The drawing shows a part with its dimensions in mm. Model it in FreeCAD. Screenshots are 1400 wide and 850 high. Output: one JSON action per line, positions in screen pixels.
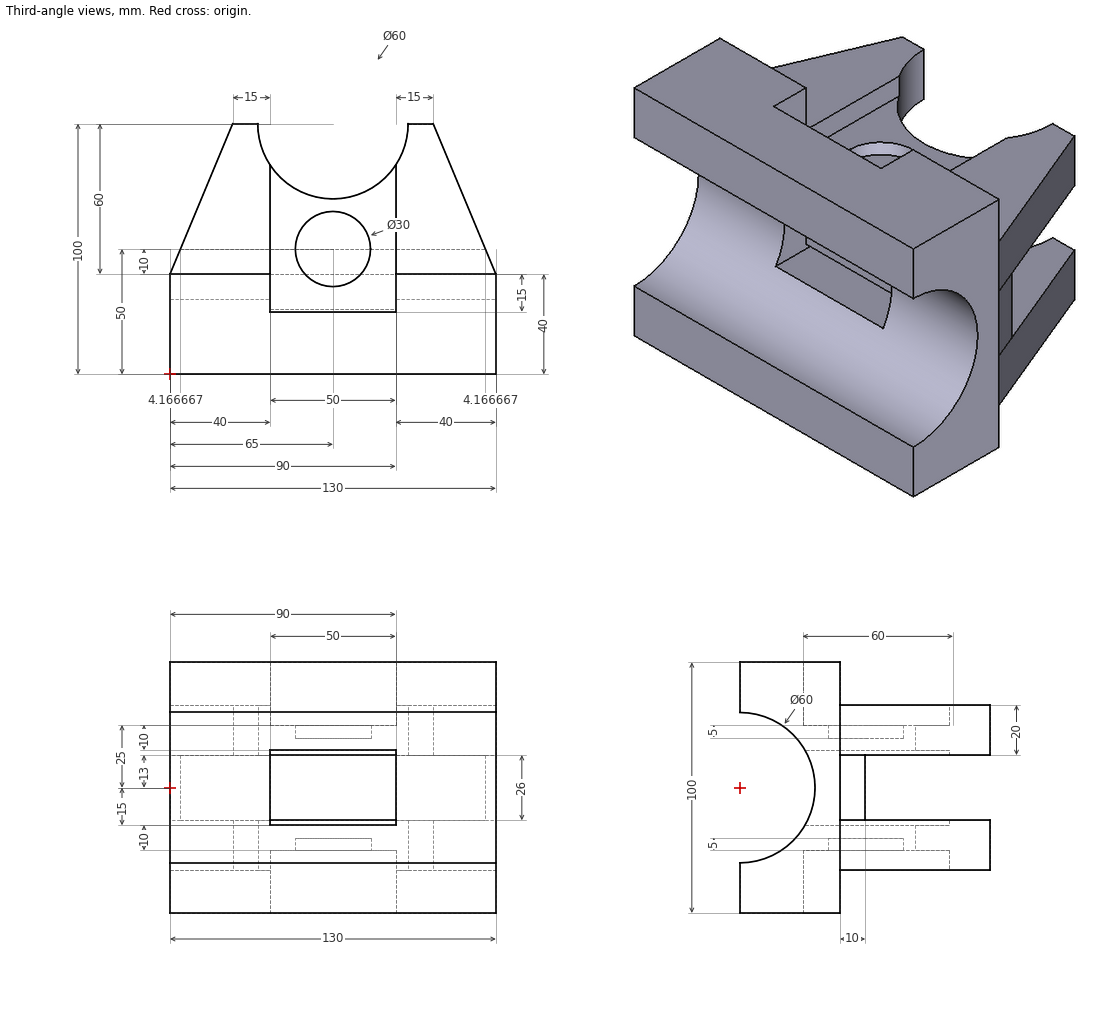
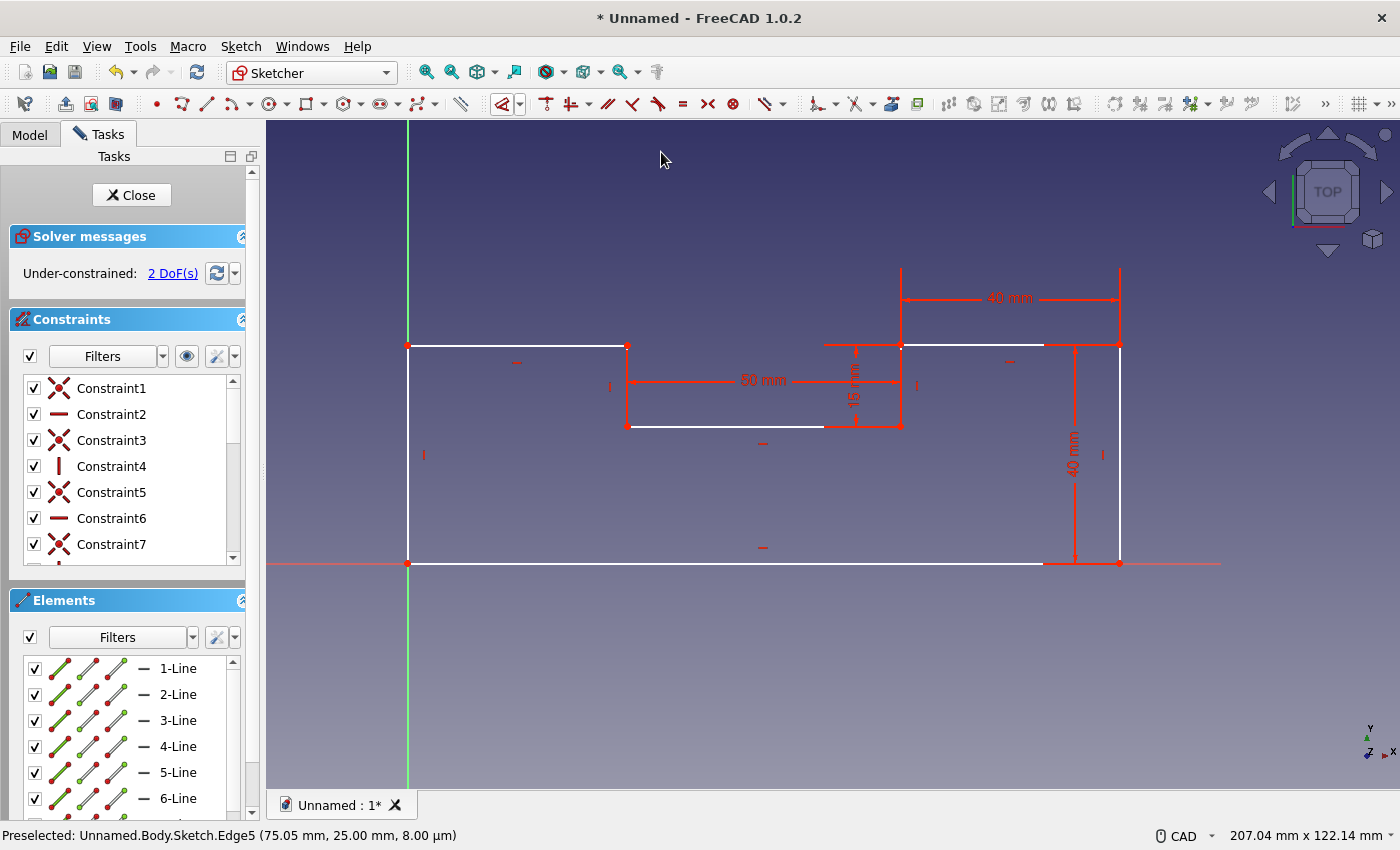
{"action": "left_click", "coordinate": [627, 403]}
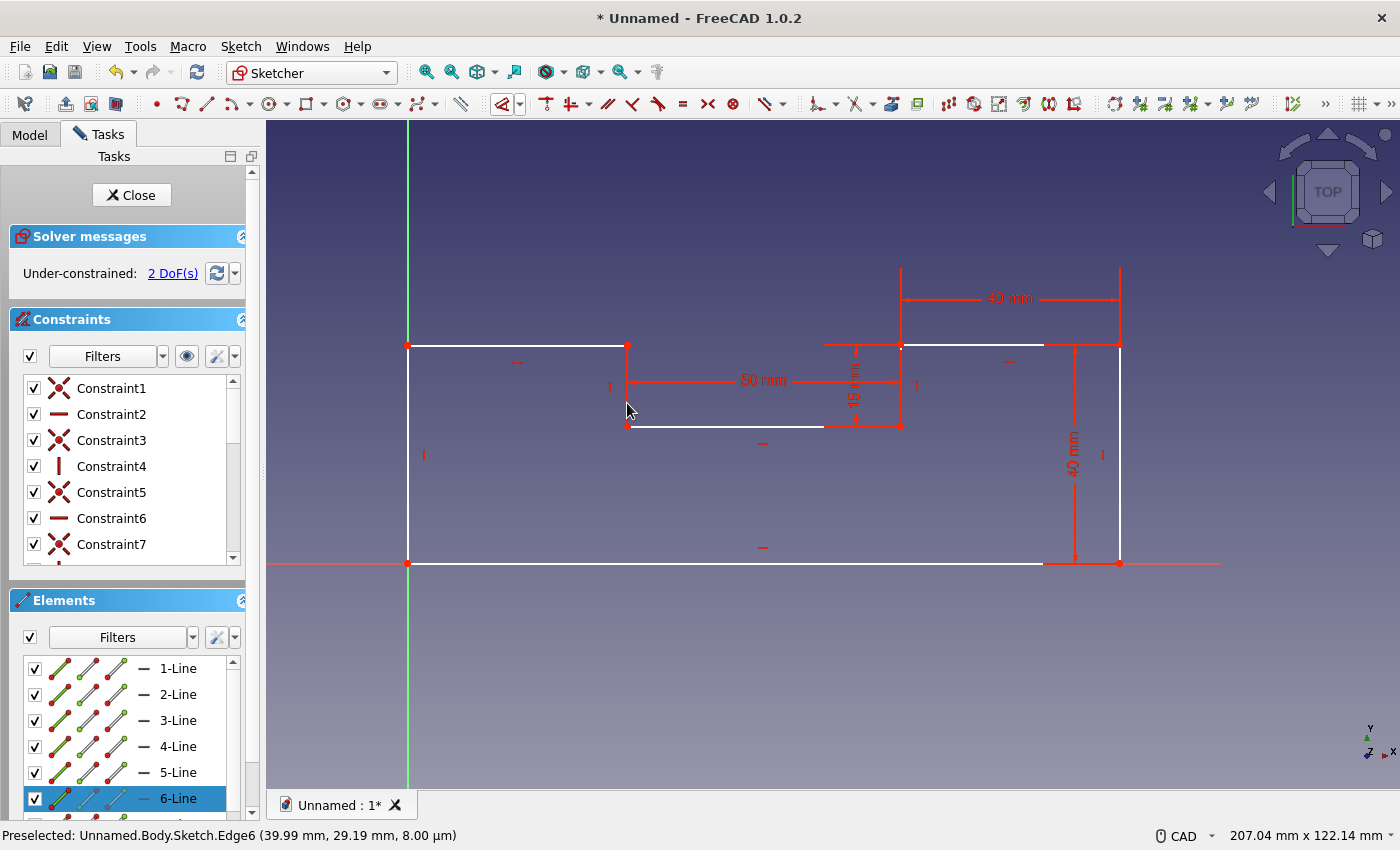
{"action": "left_click", "coordinate": [520, 104]}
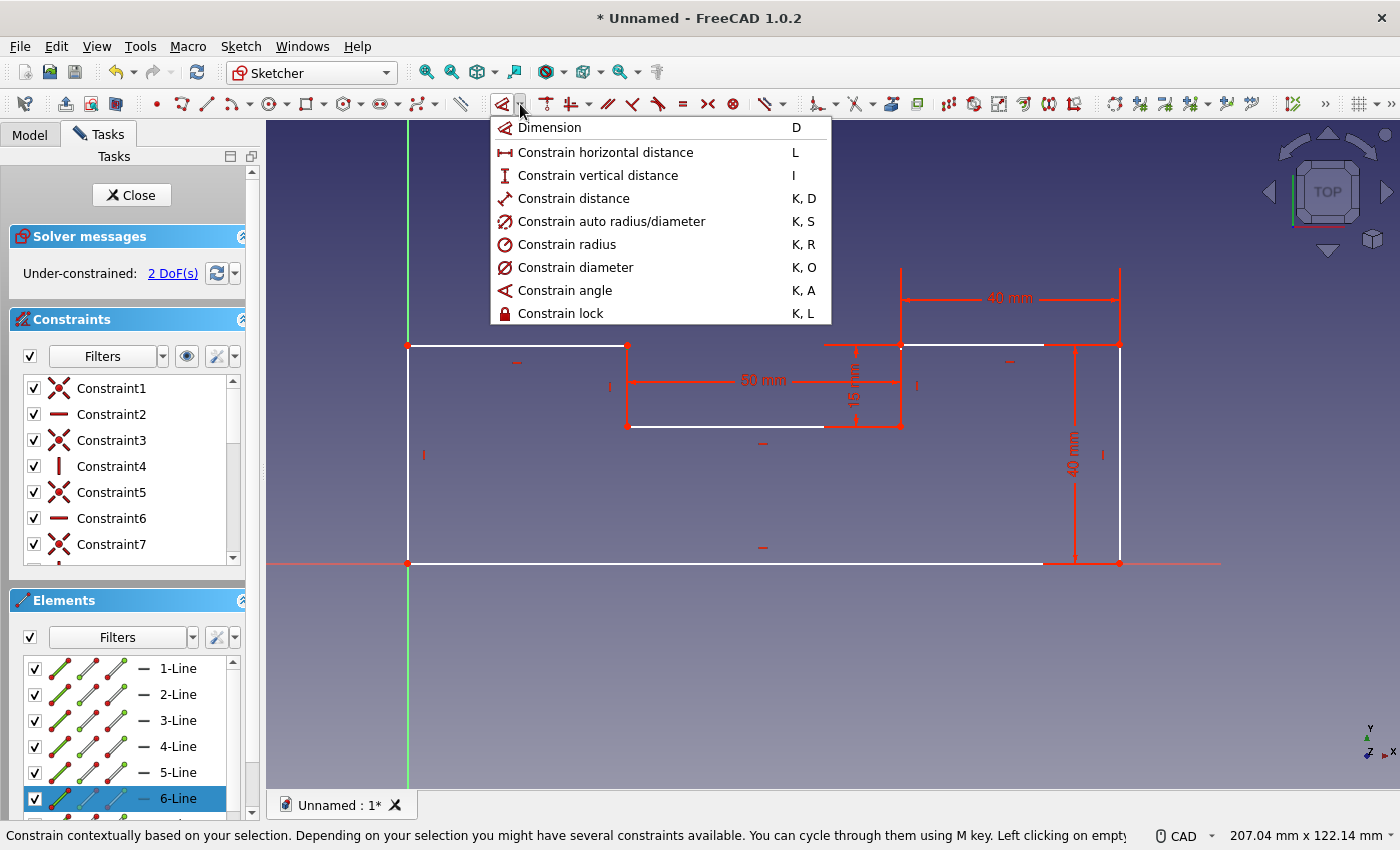
{"action": "left_click", "coordinate": [661, 176]}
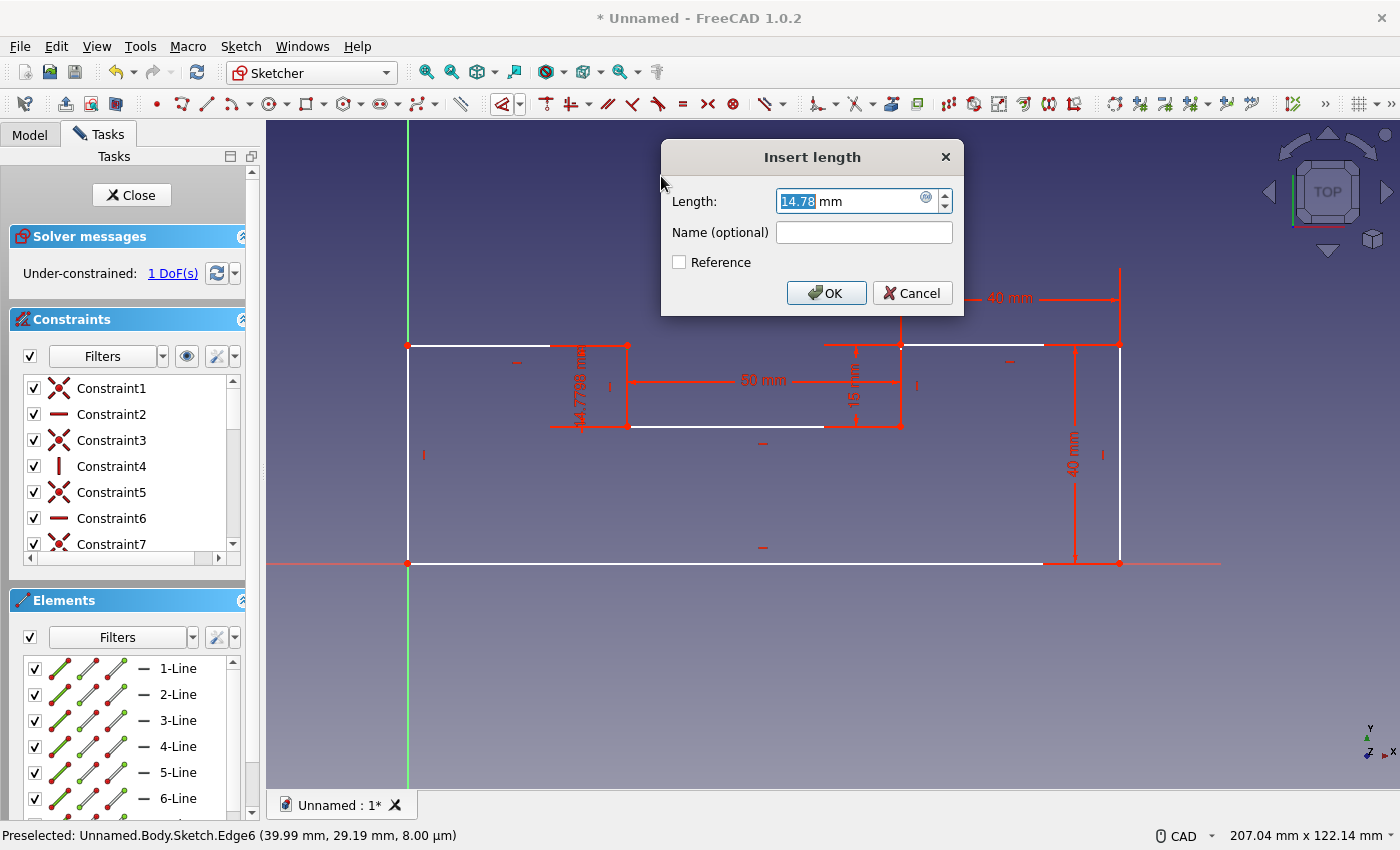
{"action": "type", "text": "15"}
{"action": "key", "text": "Return"}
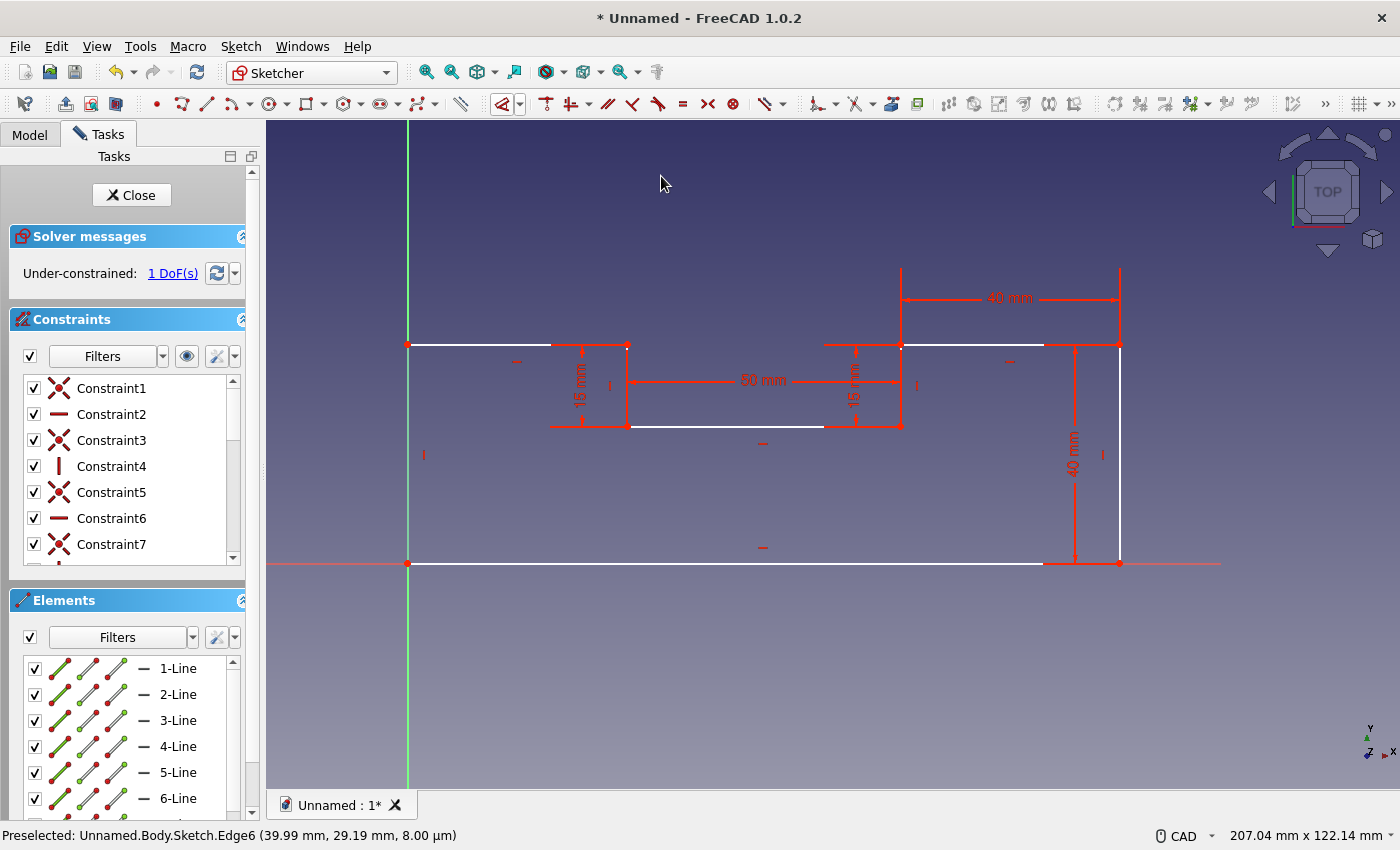
{"action": "left_click", "coordinate": [561, 345]}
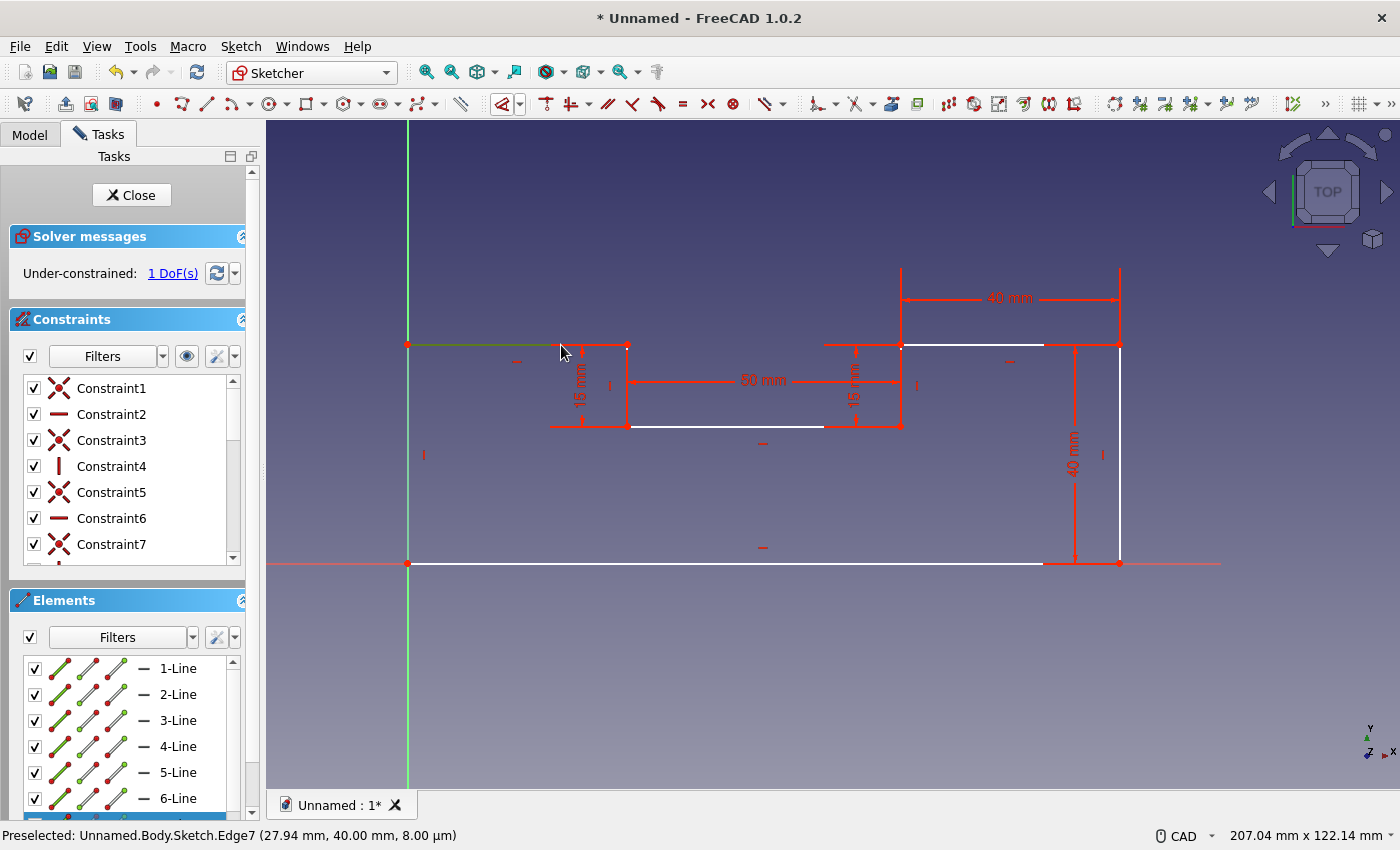
{"action": "left_click", "coordinate": [520, 104]}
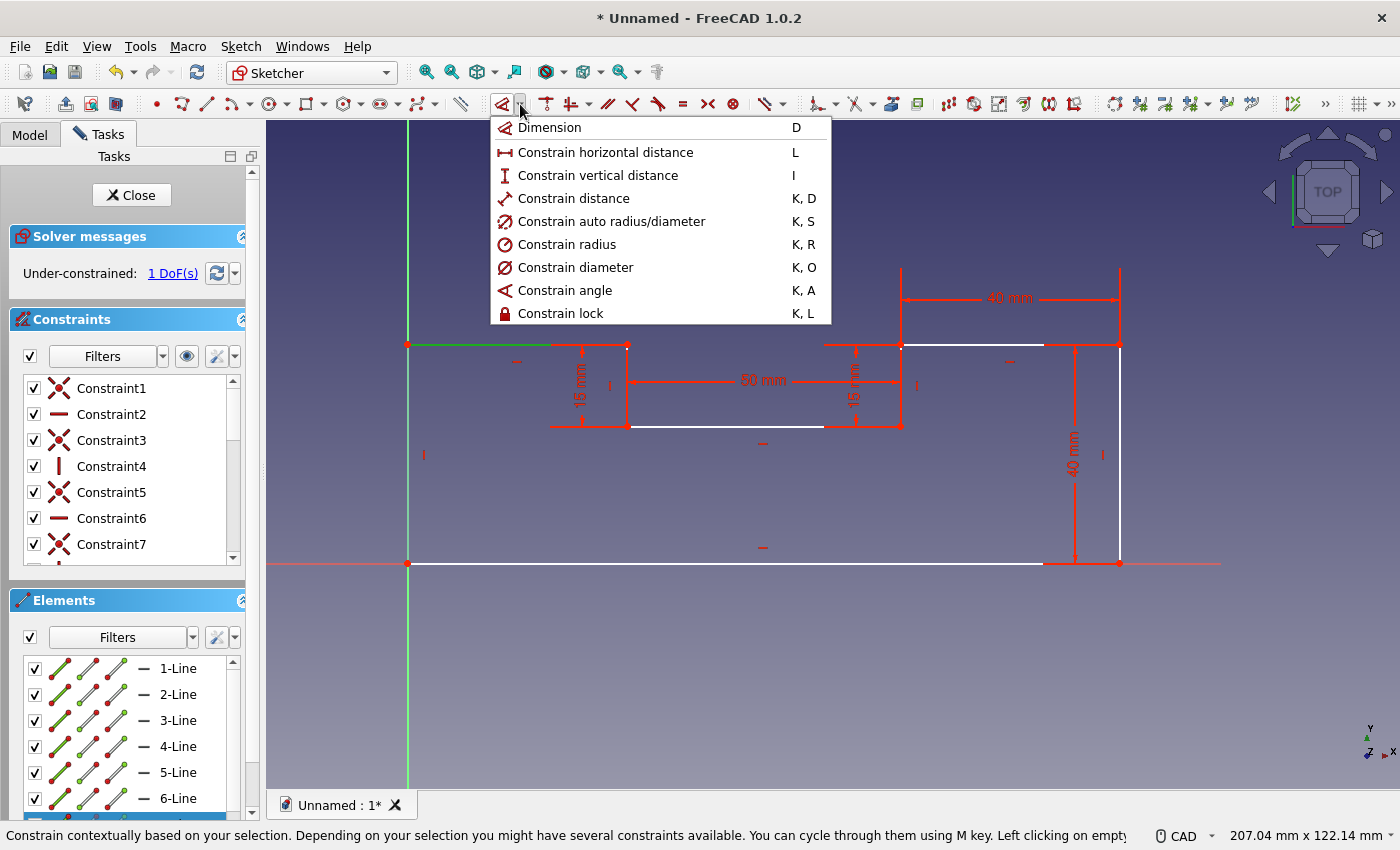
{"action": "left_click", "coordinate": [661, 152]}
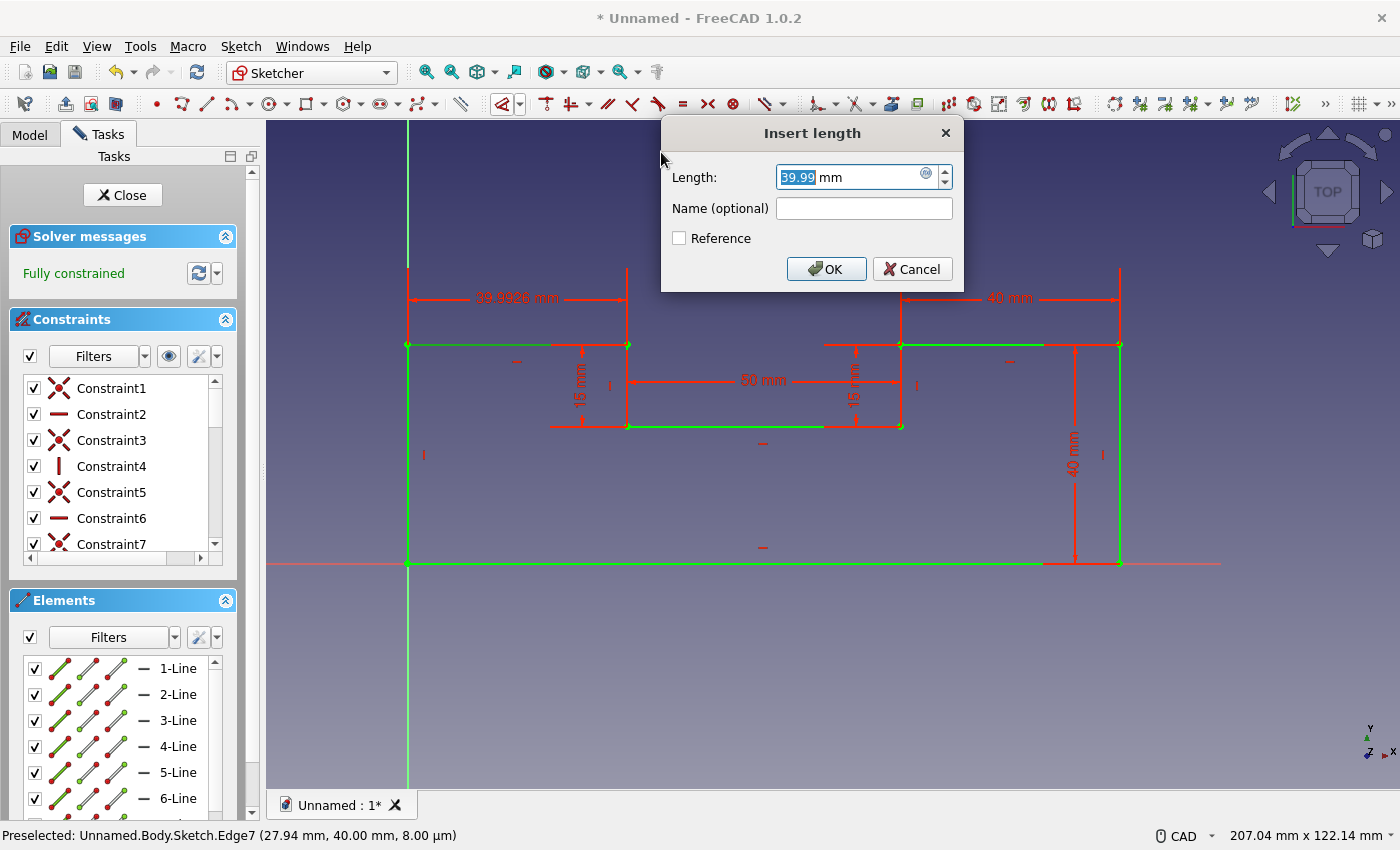
{"action": "type", "text": "40"}
{"action": "key", "text": "Return"}